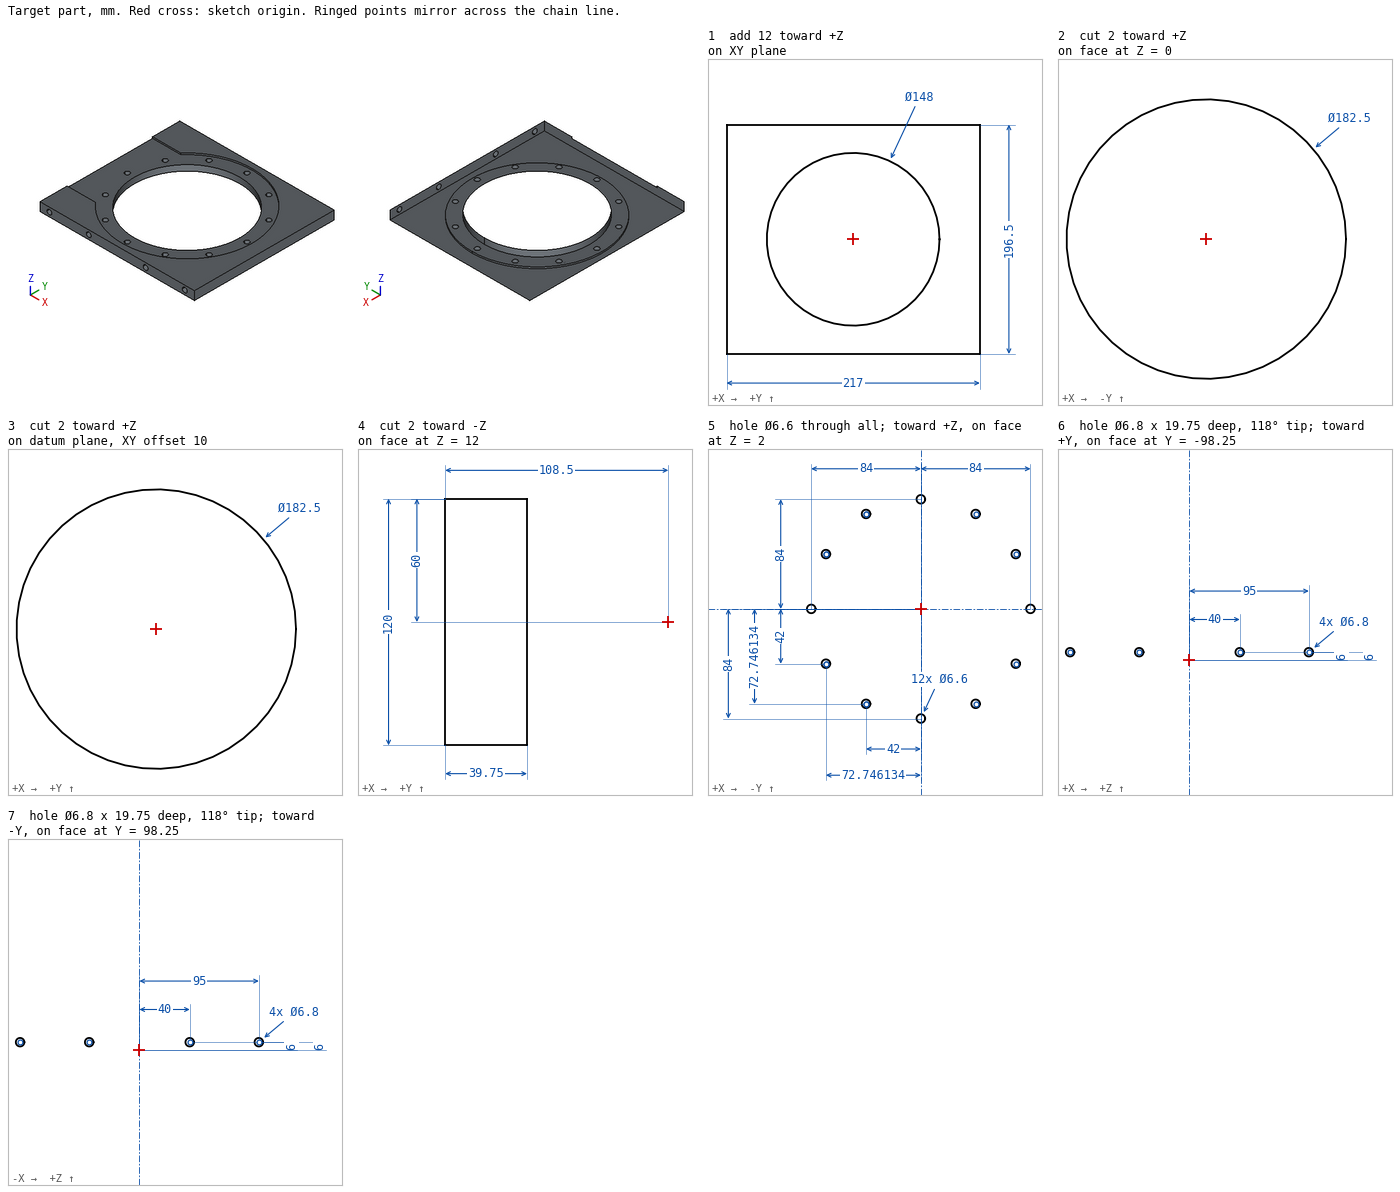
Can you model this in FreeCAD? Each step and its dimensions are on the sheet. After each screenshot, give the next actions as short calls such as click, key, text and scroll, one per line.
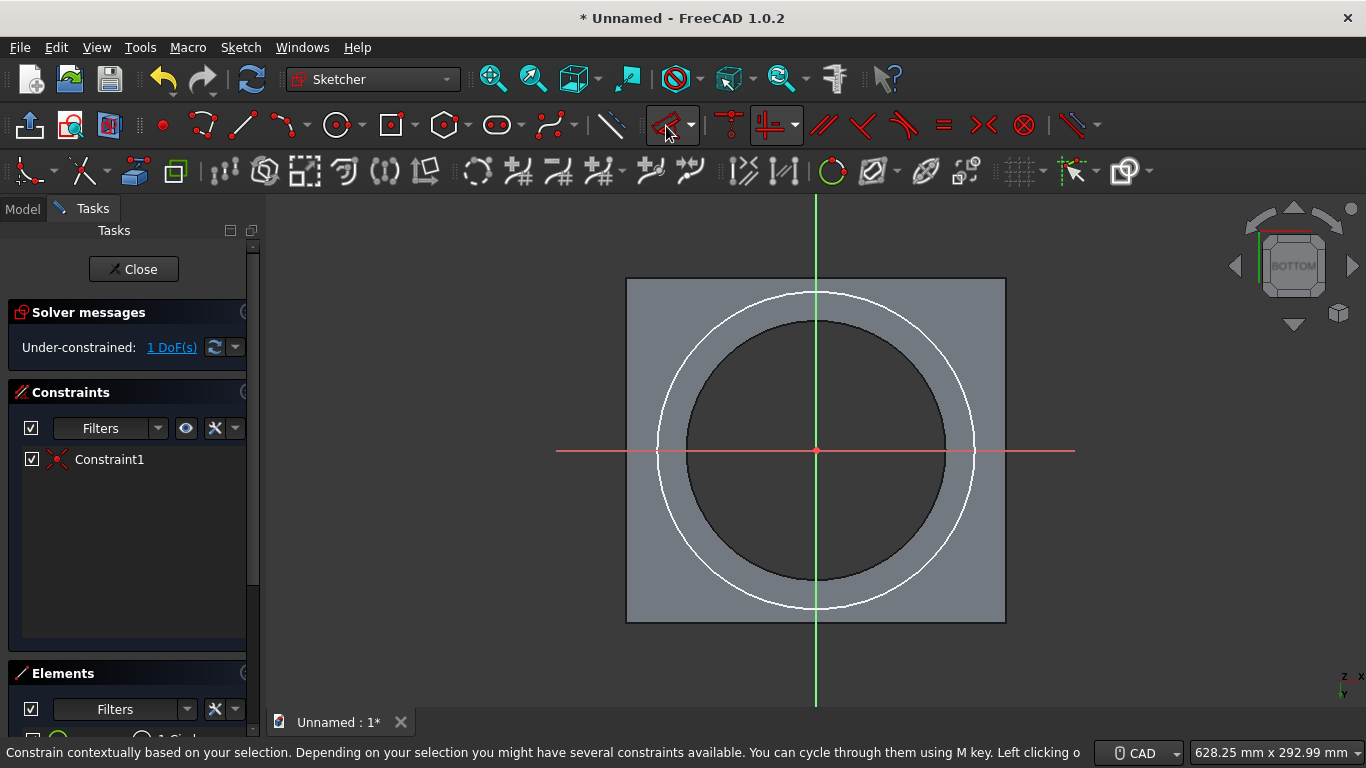
click(928, 338)
click(951, 315)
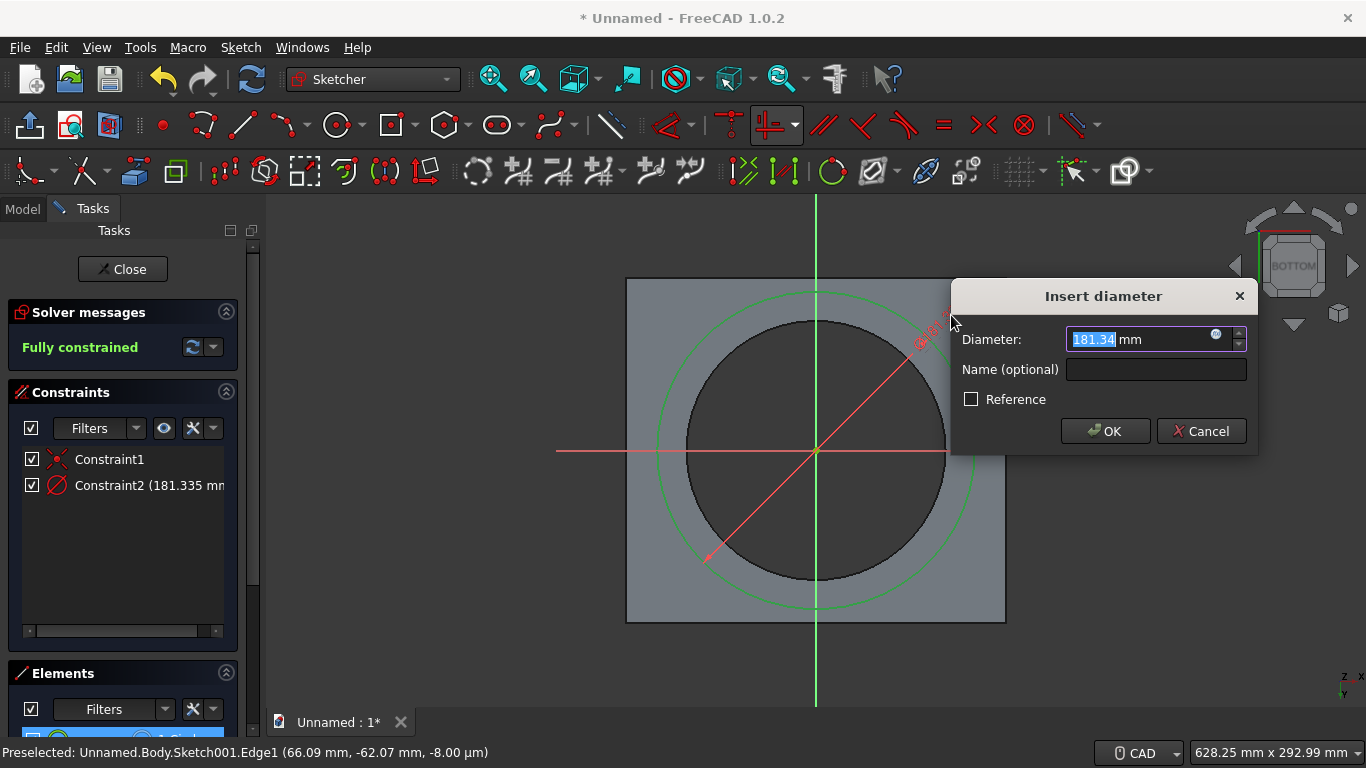
text(182.5)
key(Return)
key(Escape)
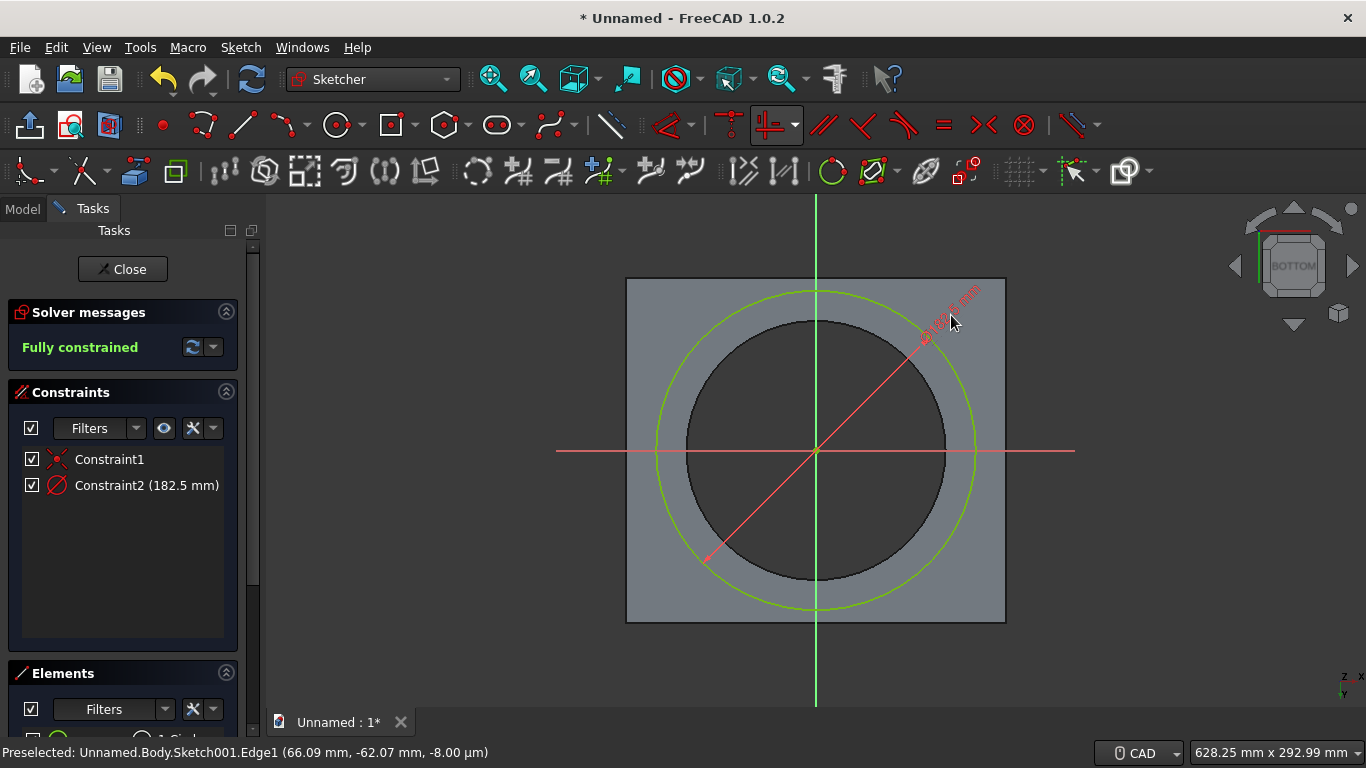
click(123, 269)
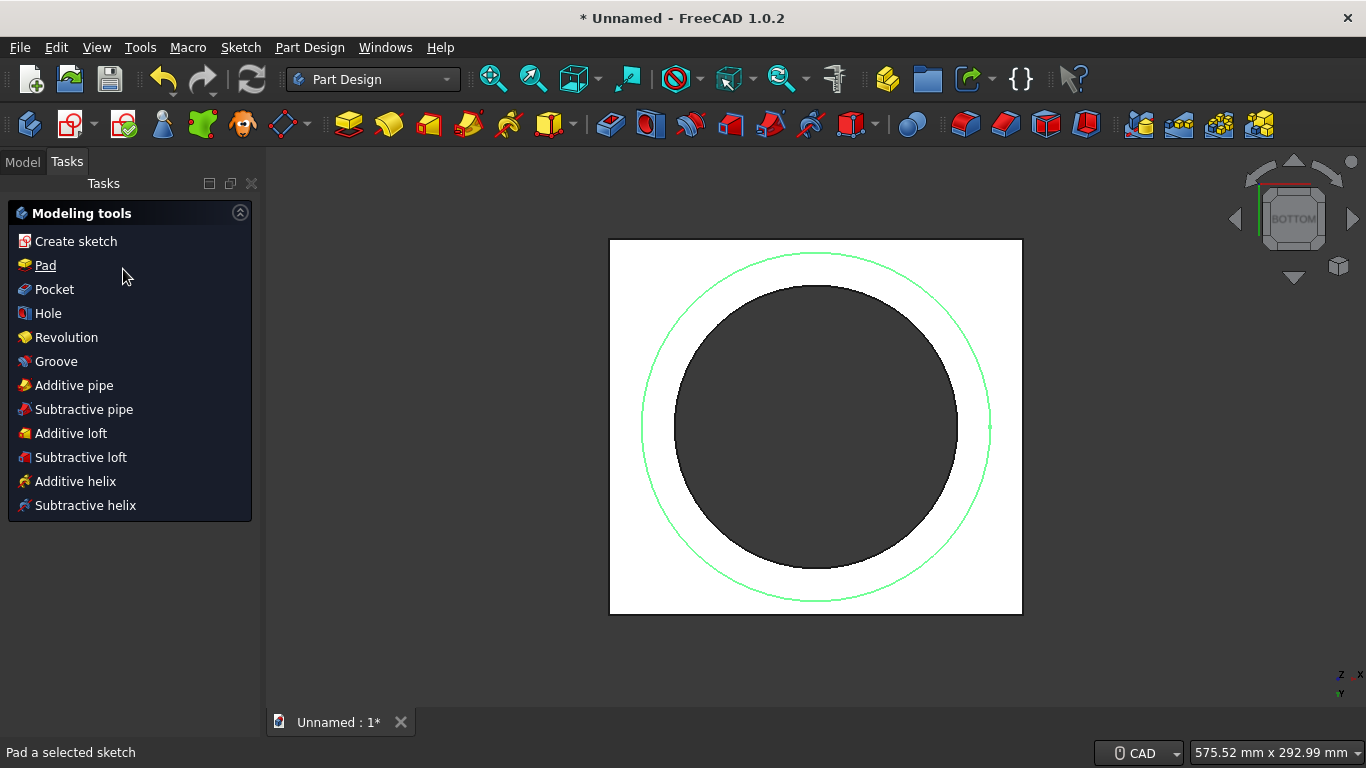
click(612, 124)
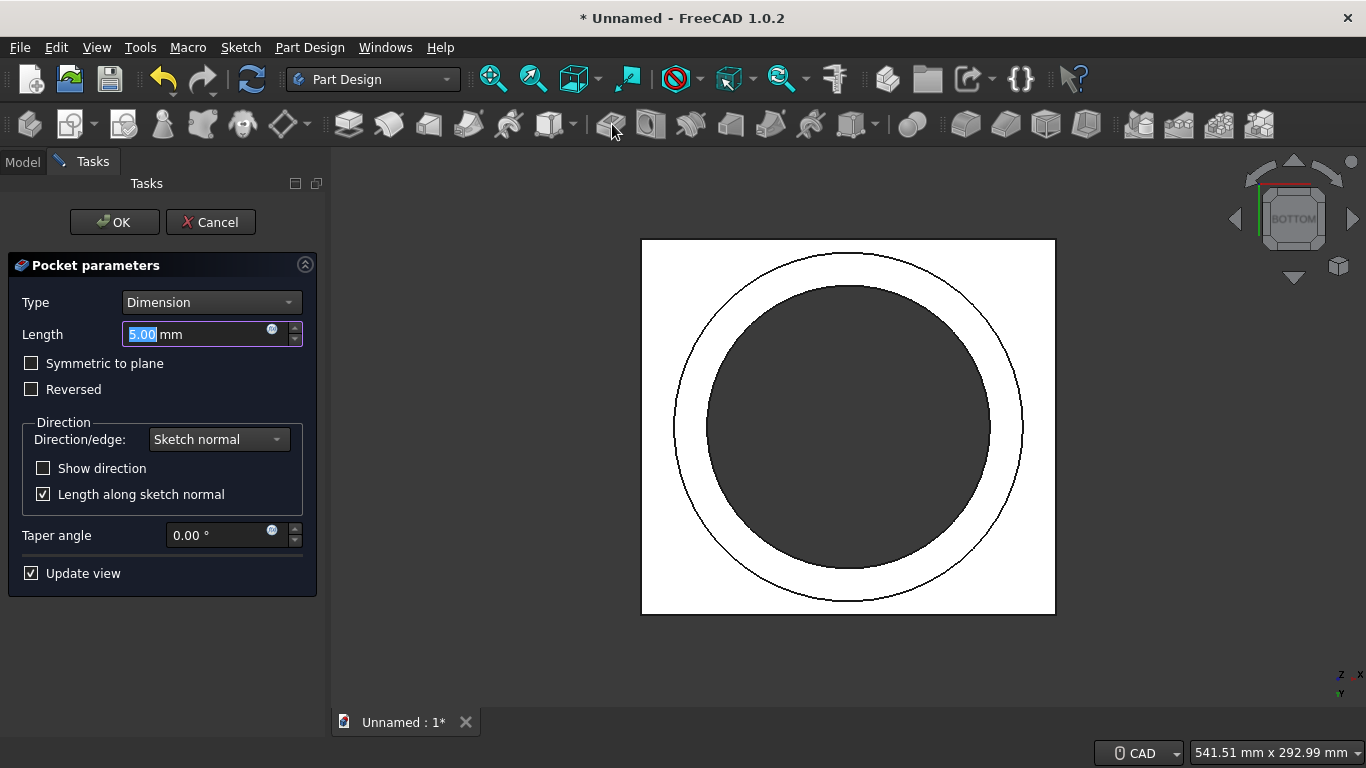
text(2)
key(Tab)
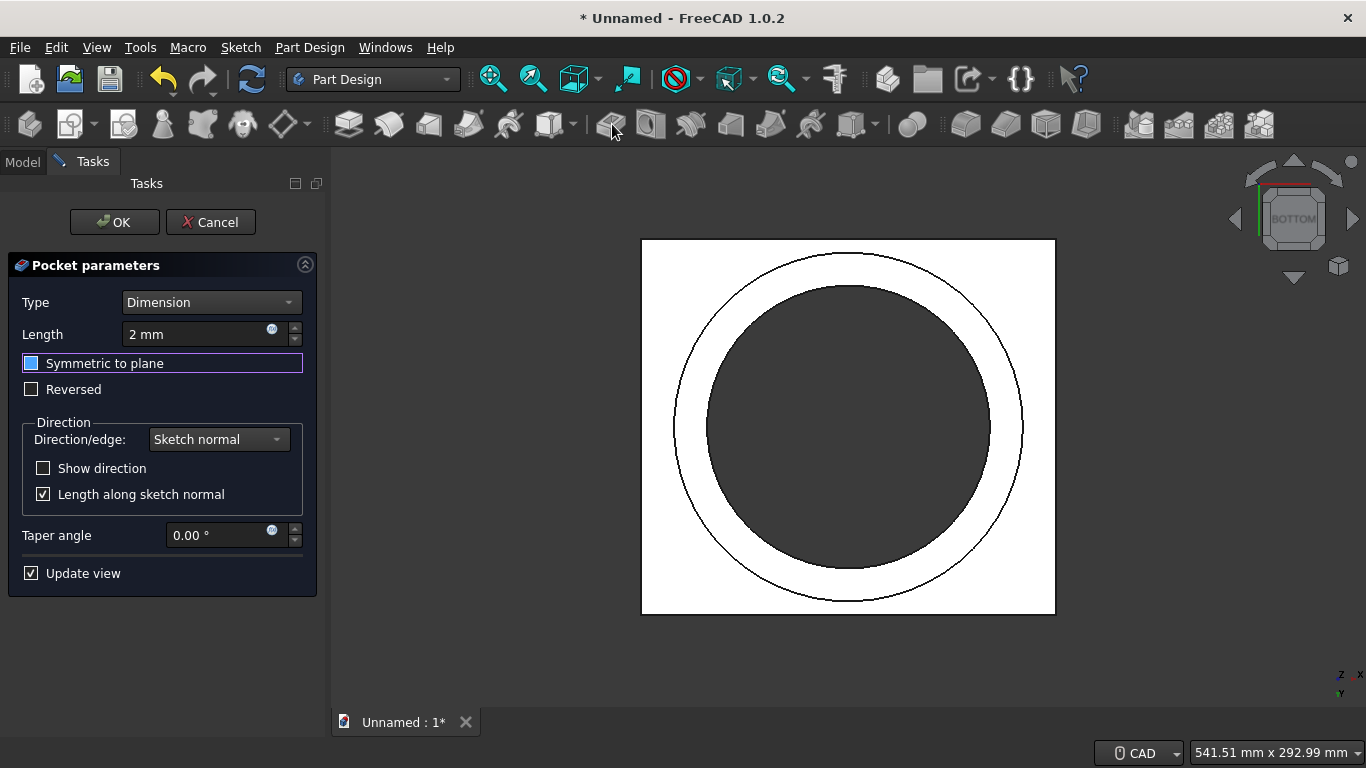
click(115, 222)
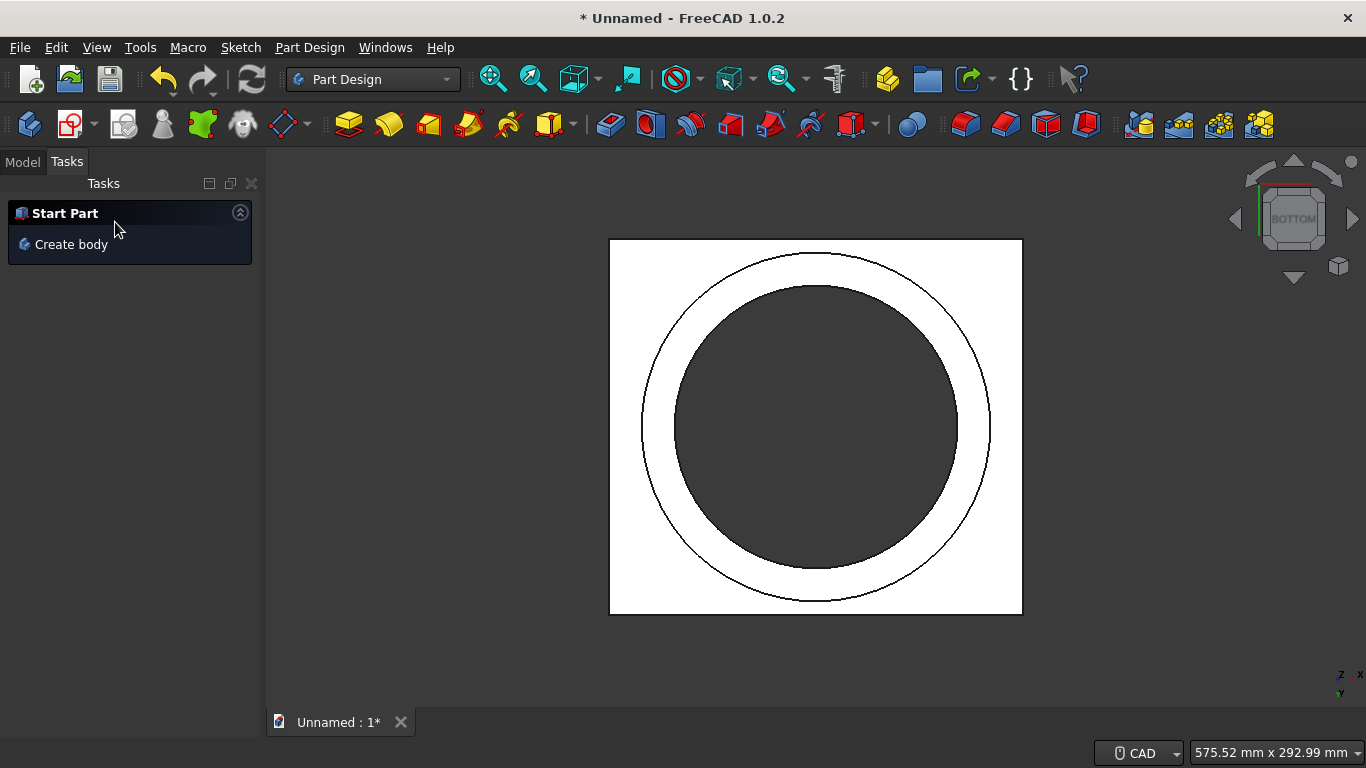
click(23, 161)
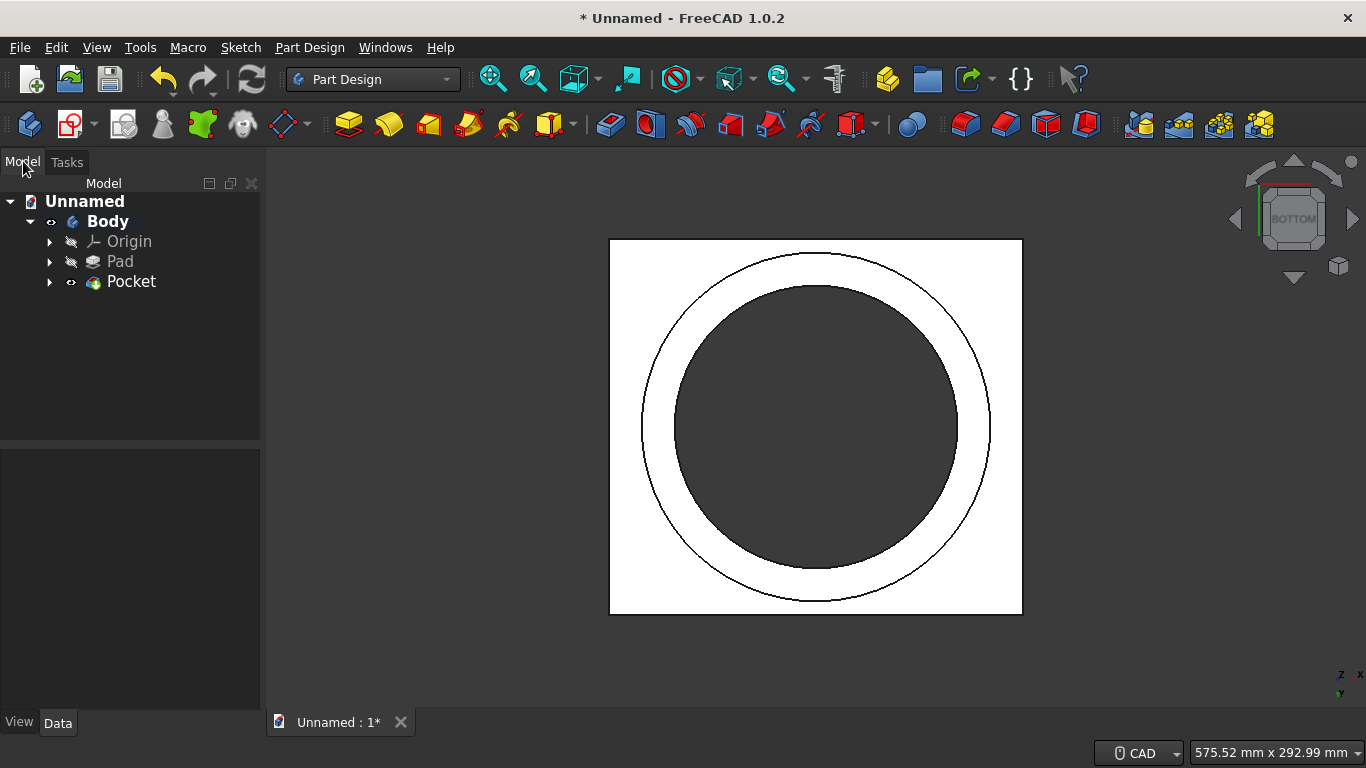
click(50, 242)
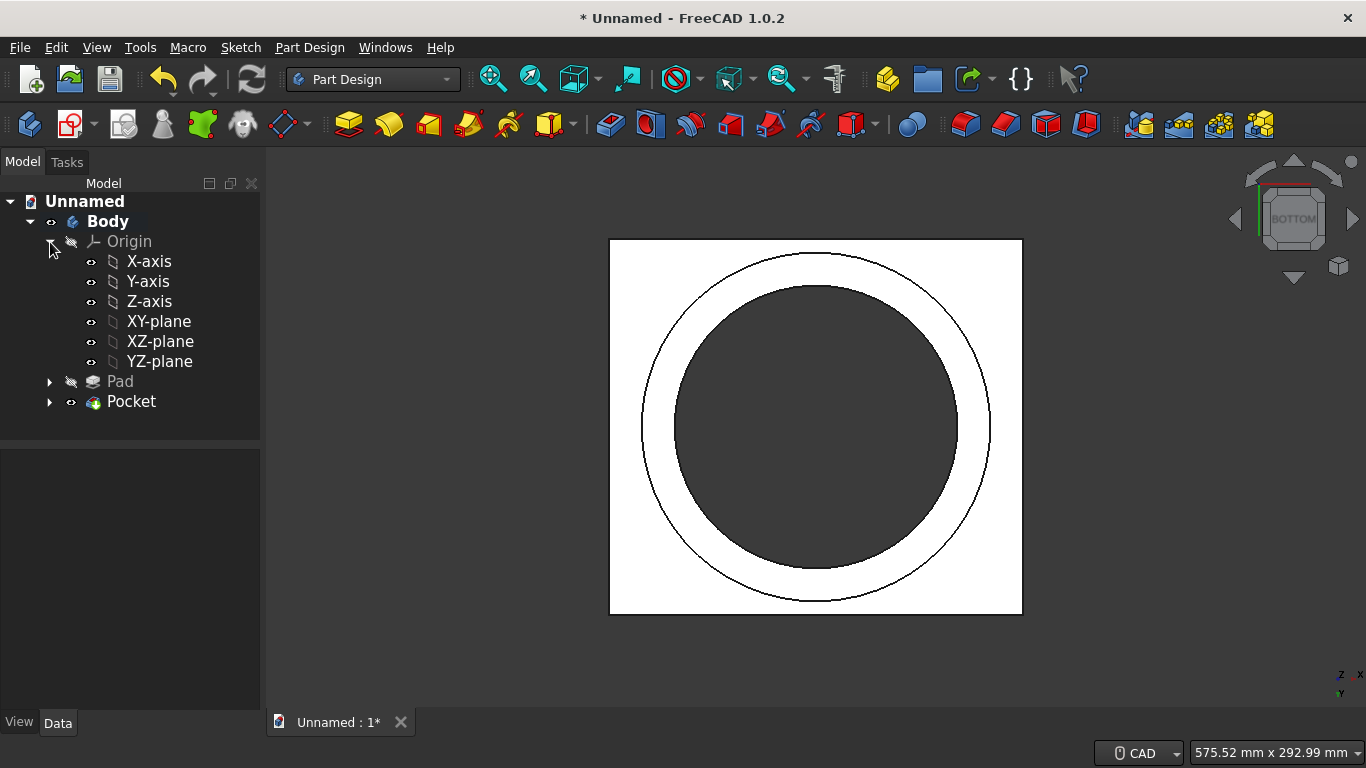
click(136, 322)